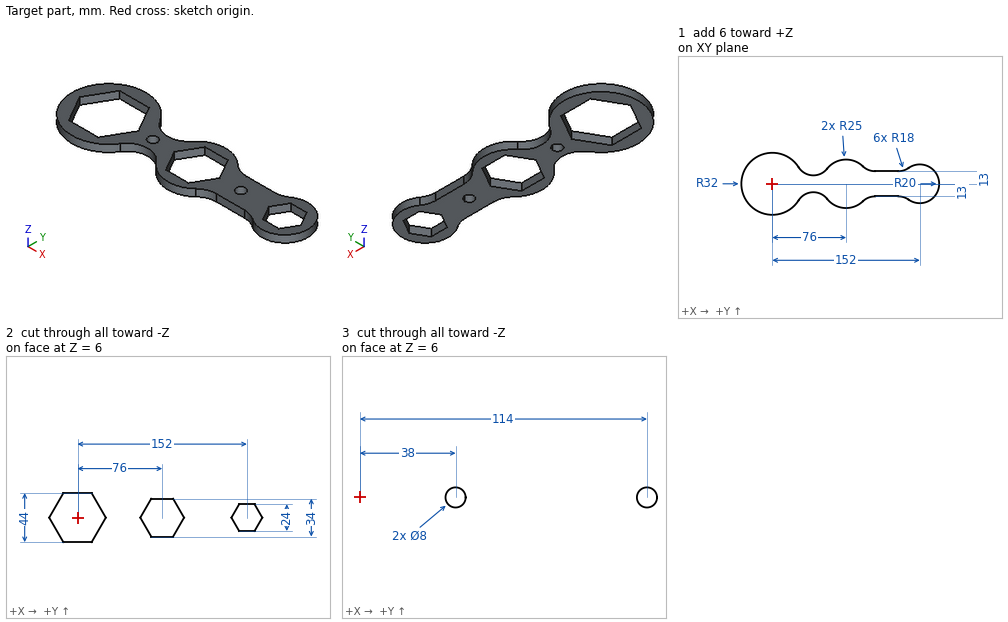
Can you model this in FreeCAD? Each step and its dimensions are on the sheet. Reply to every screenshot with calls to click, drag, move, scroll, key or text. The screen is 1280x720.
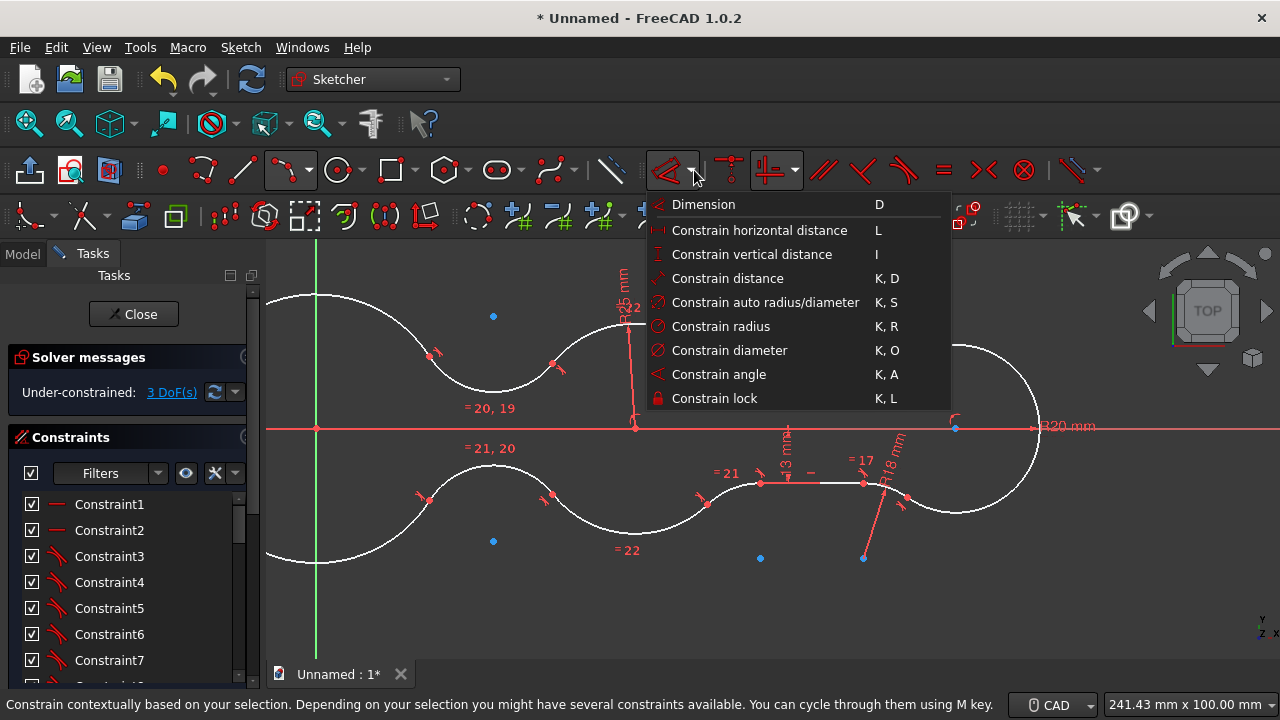
click(799, 254)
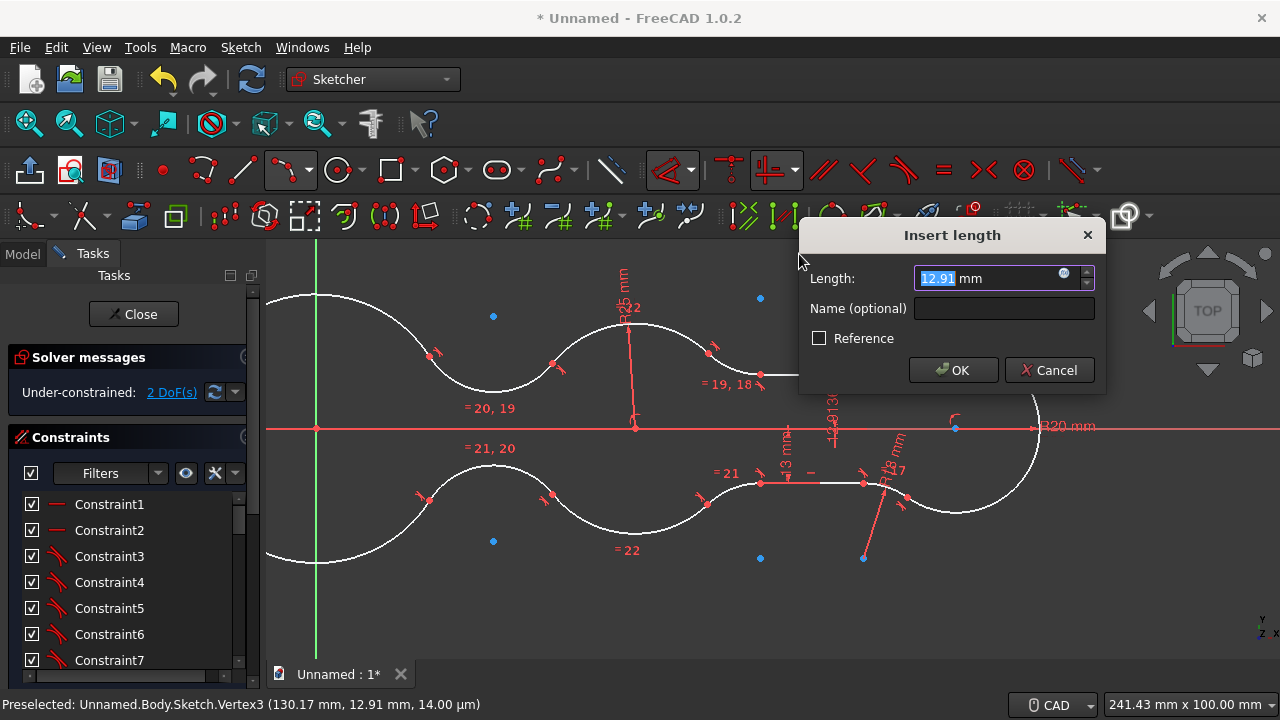
text(13)
key(Return)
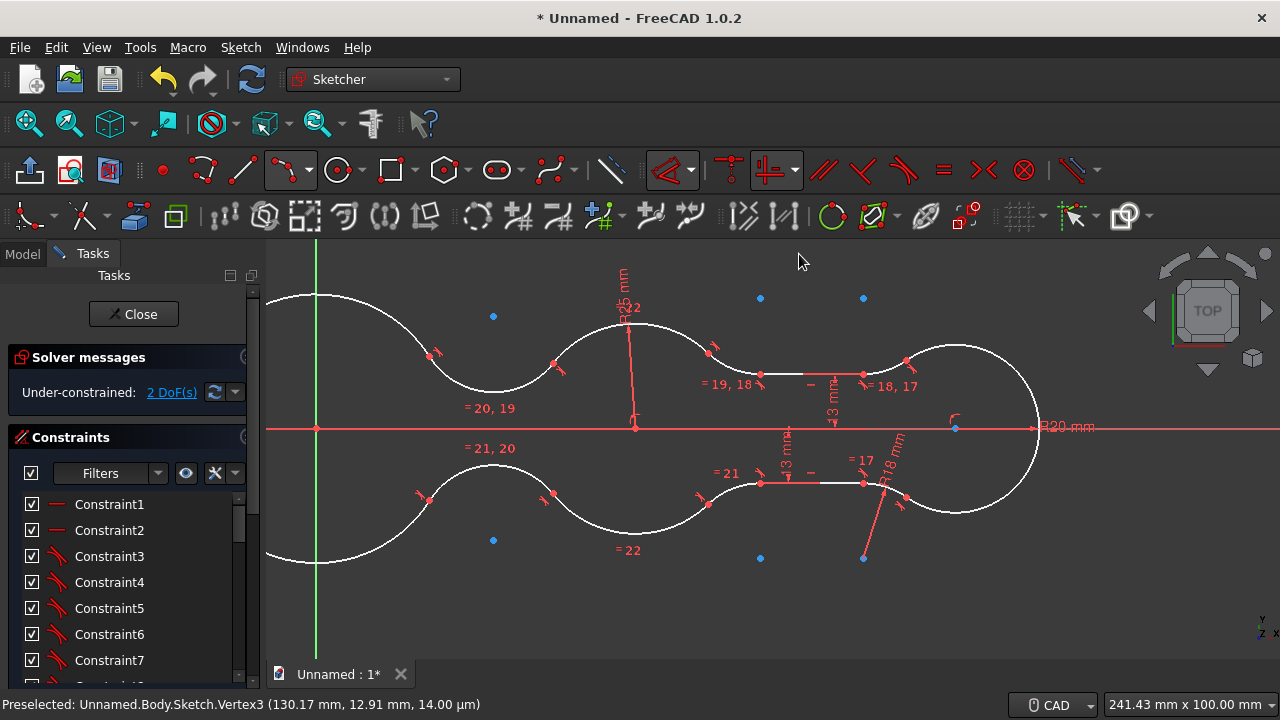
click(635, 429)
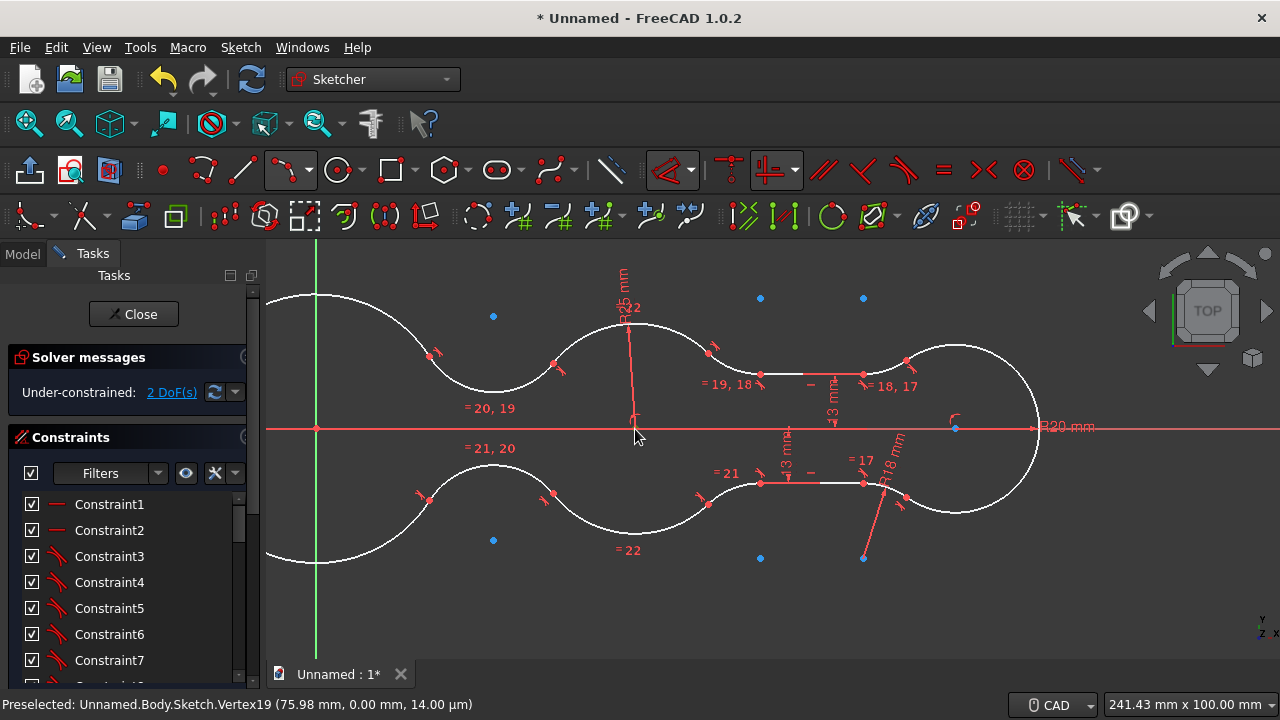
click(694, 170)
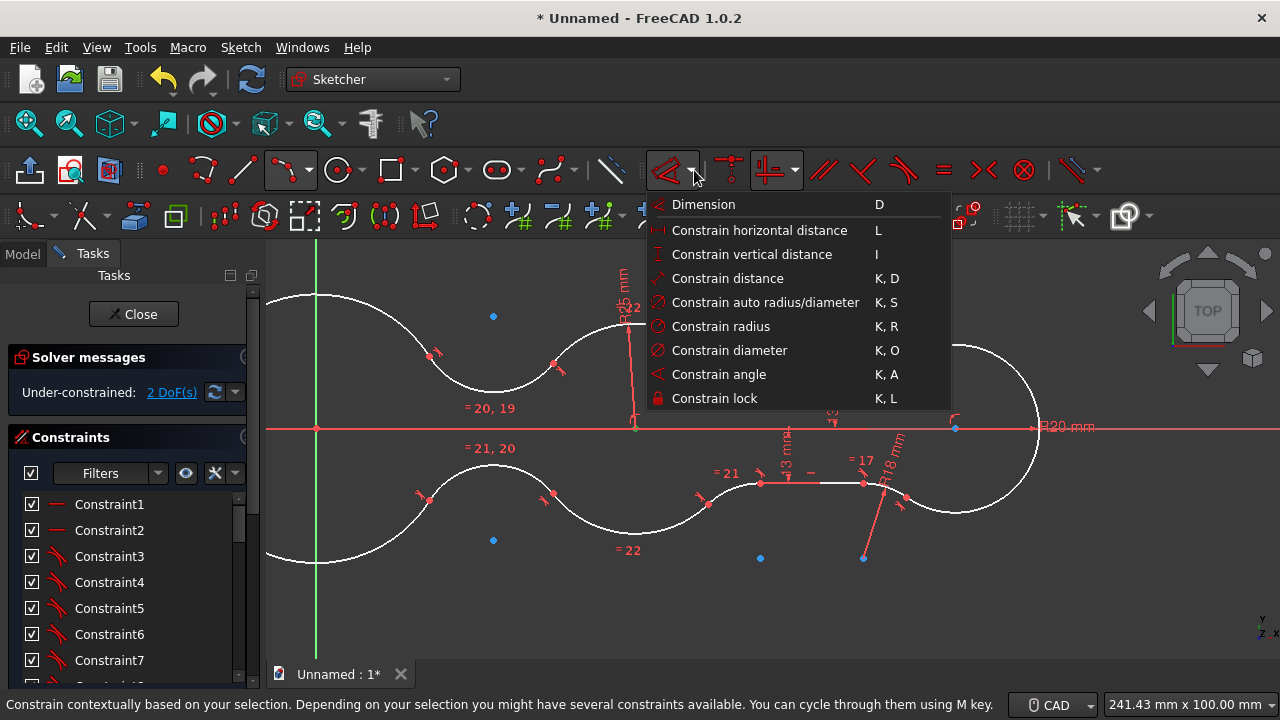
click(799, 230)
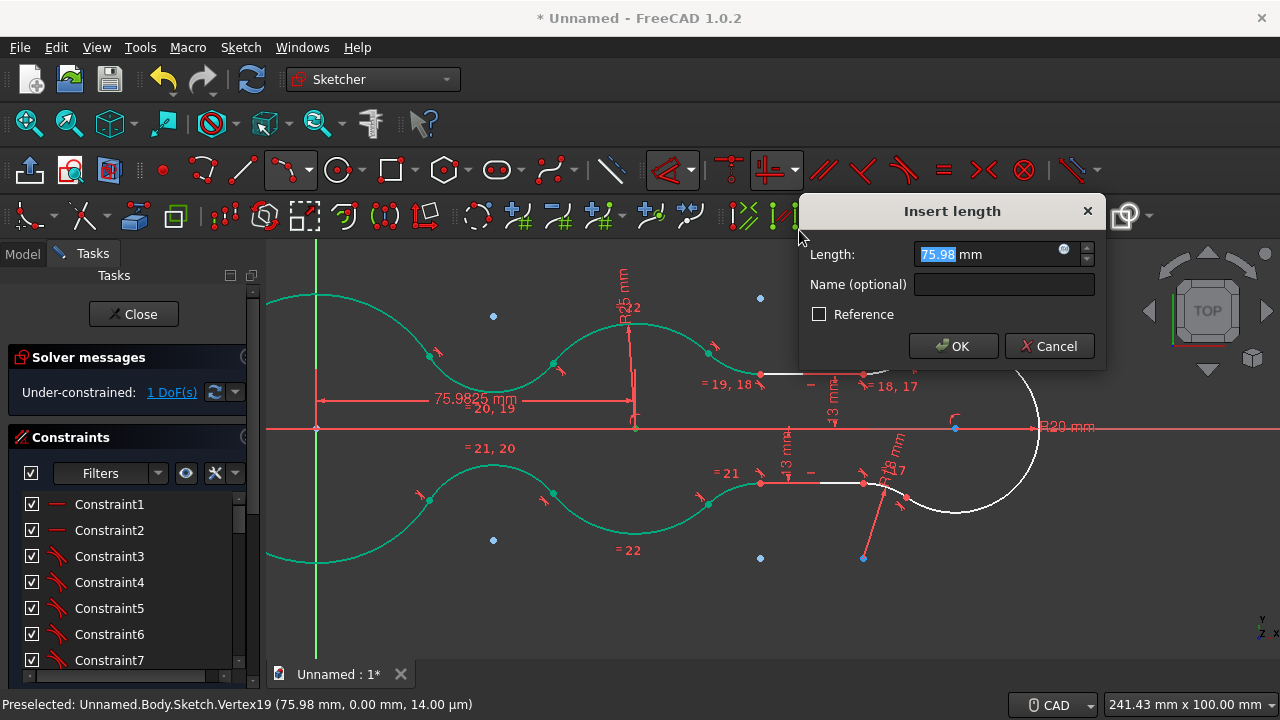
text(76)
key(Return)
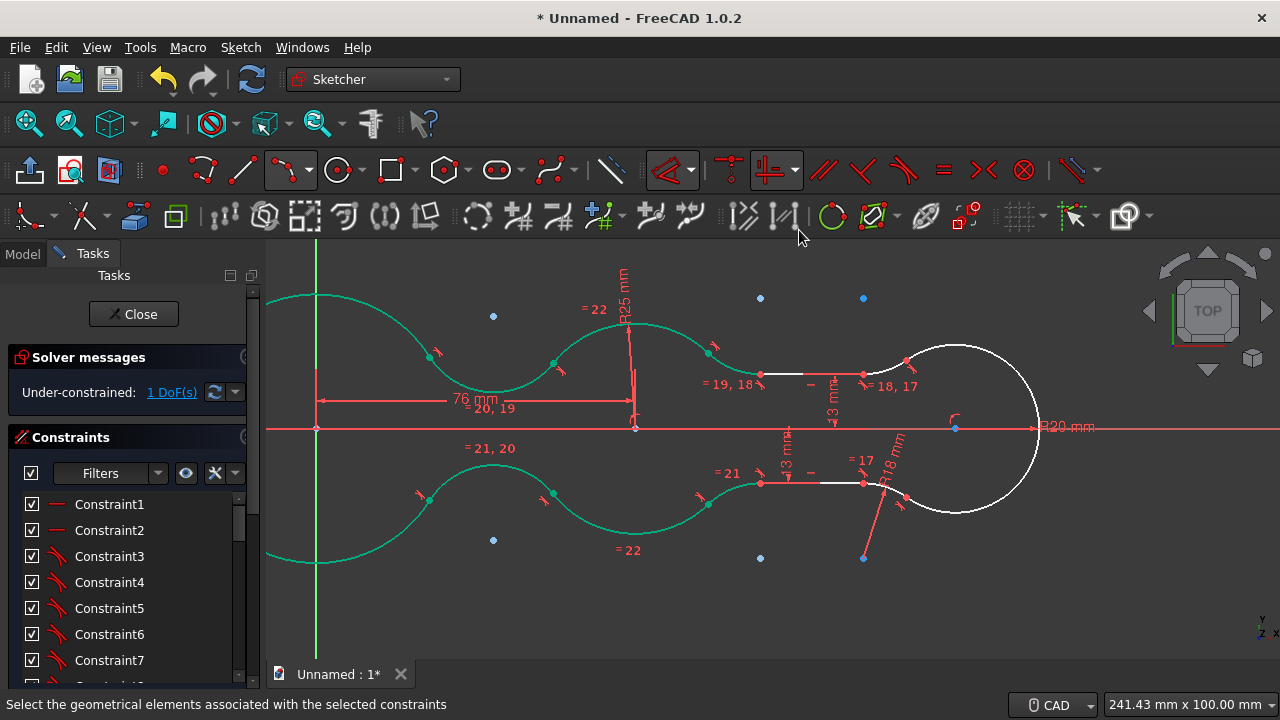
click(955, 429)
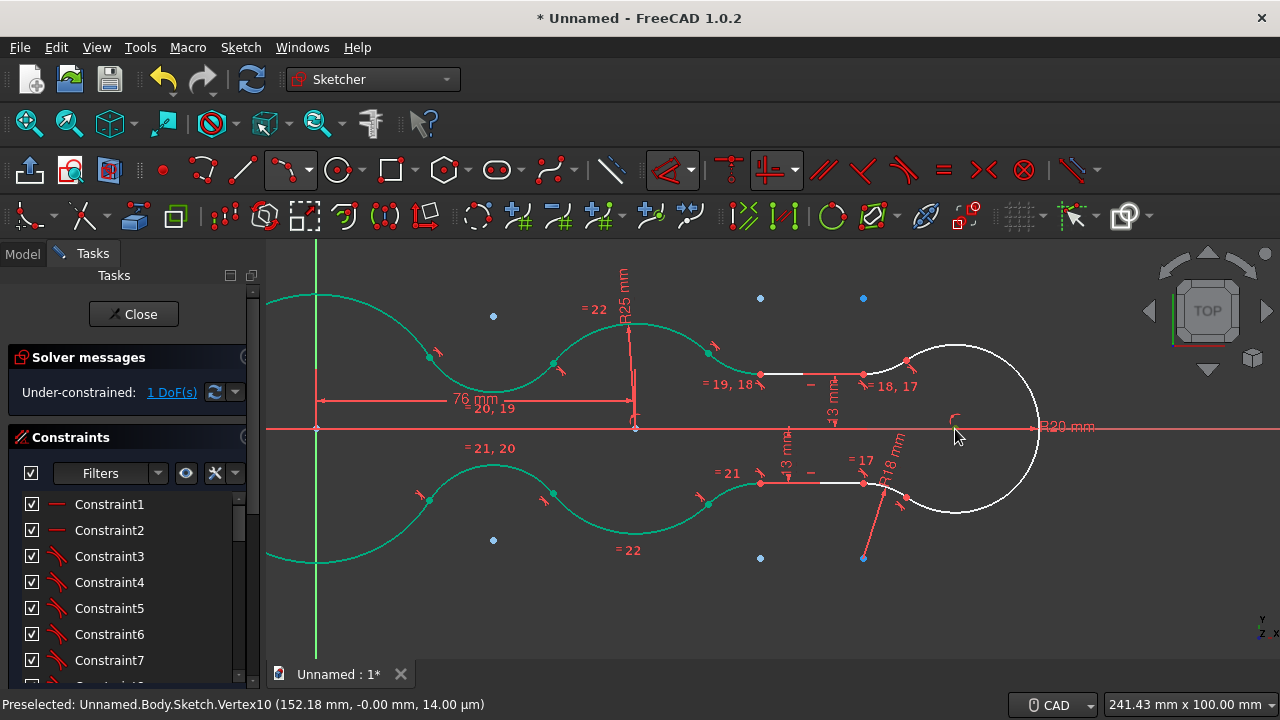
key(l)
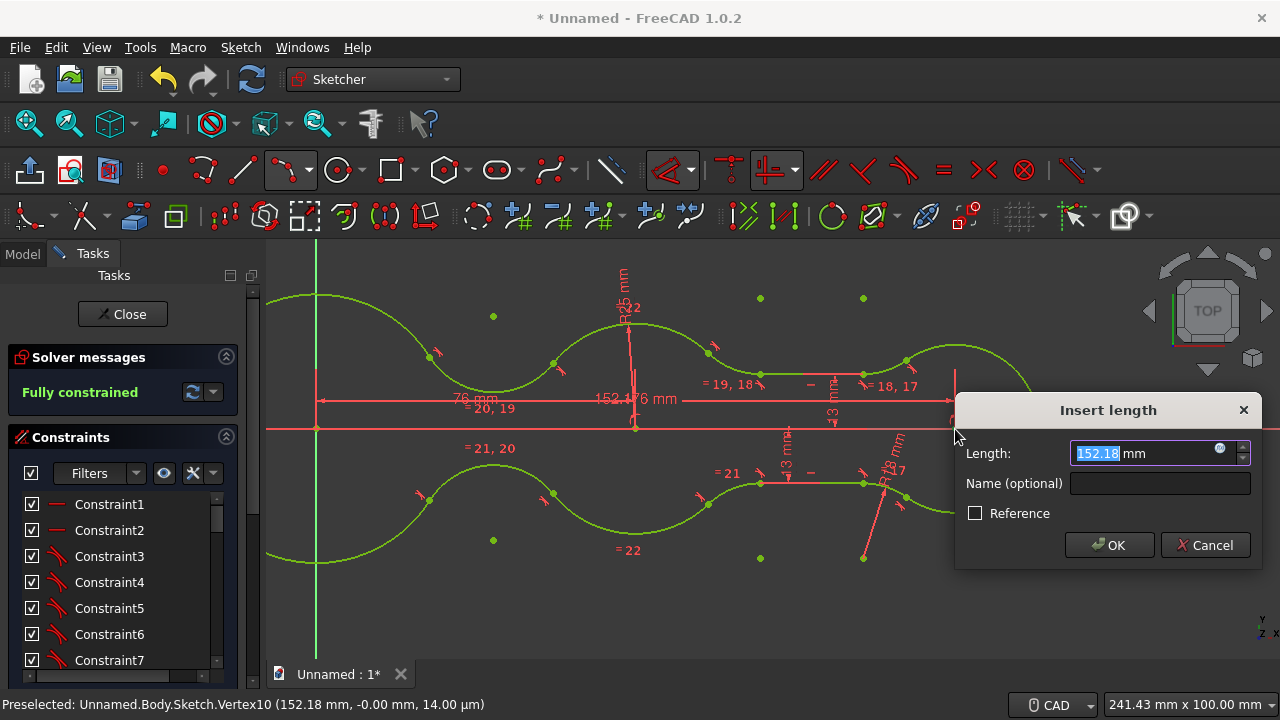
text(152)
key(Return)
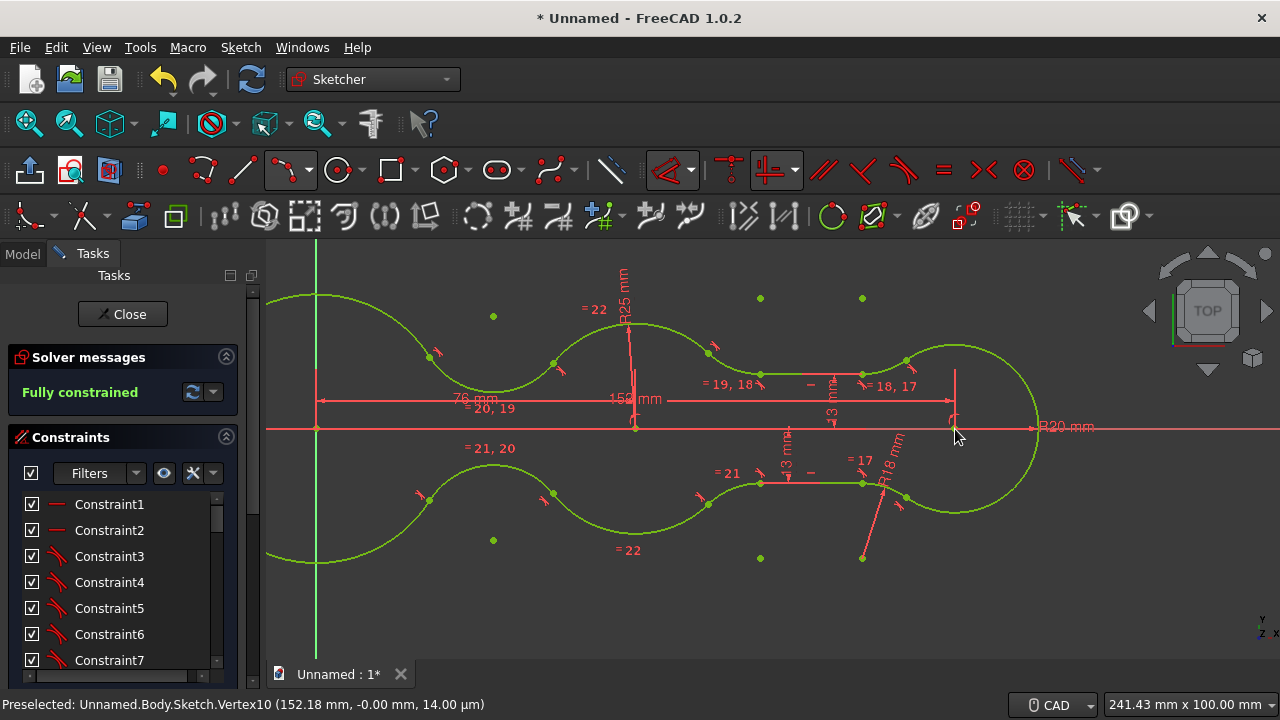
click(123, 314)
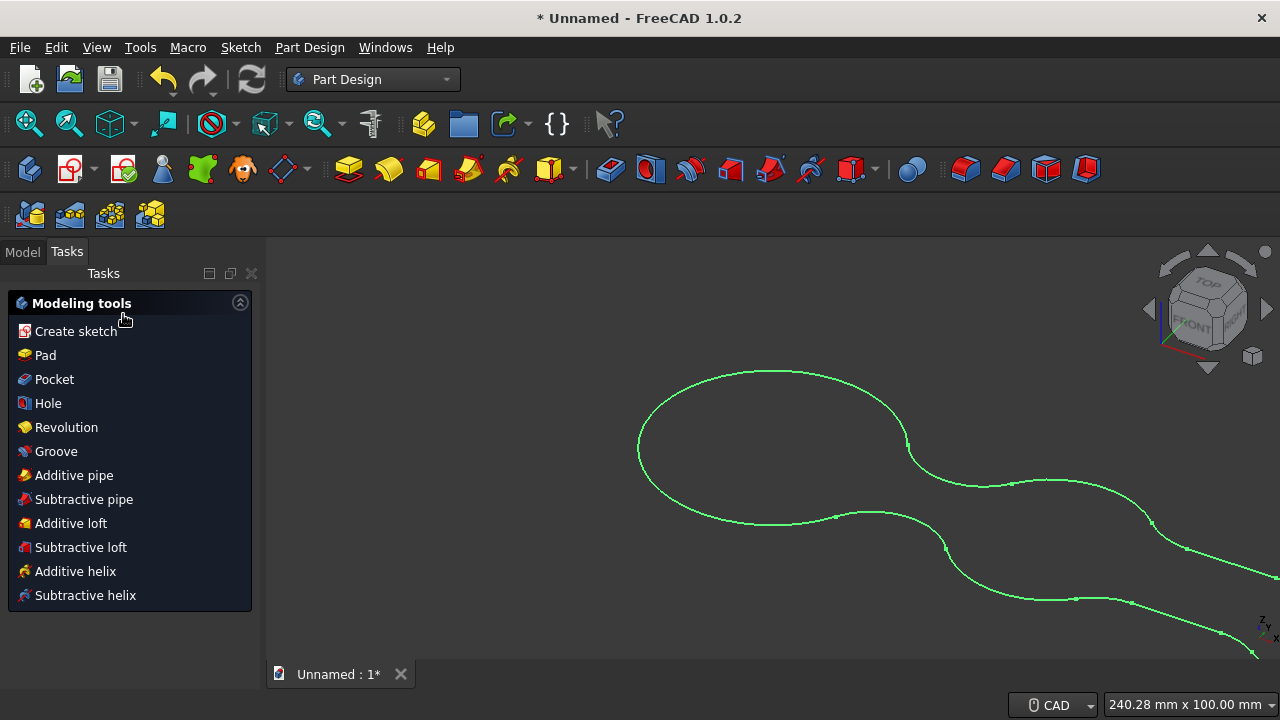
click(350, 170)